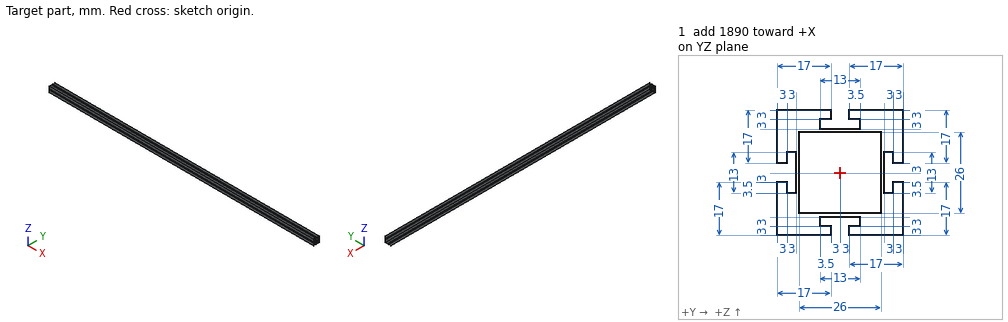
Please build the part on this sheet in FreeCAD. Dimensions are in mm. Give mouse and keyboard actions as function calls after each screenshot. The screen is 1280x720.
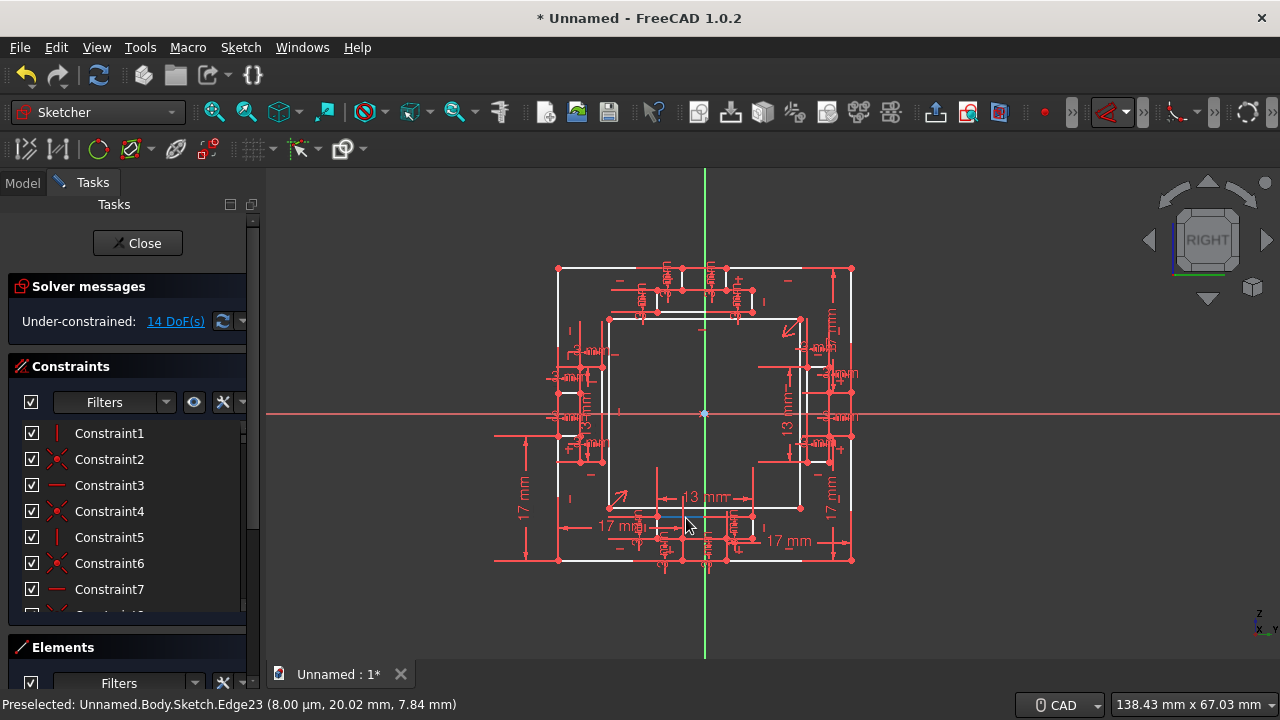
click(814, 268)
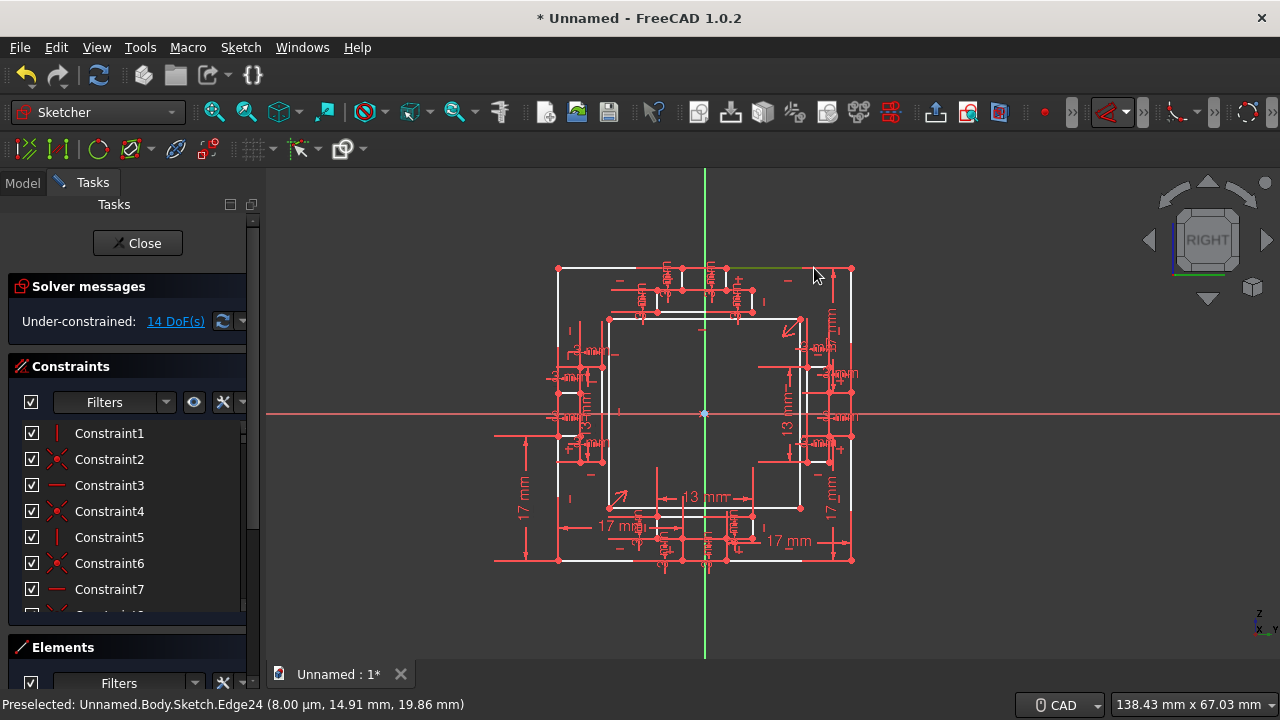
key(l)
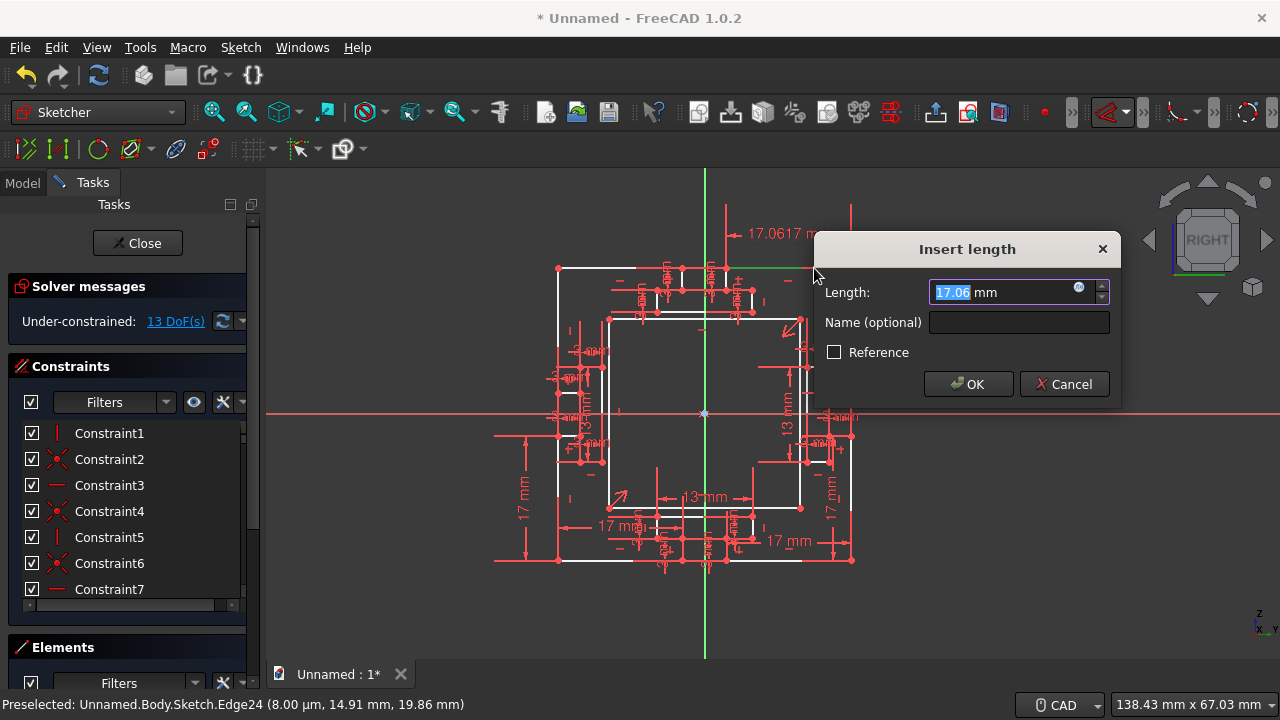
text(17)
key(Return)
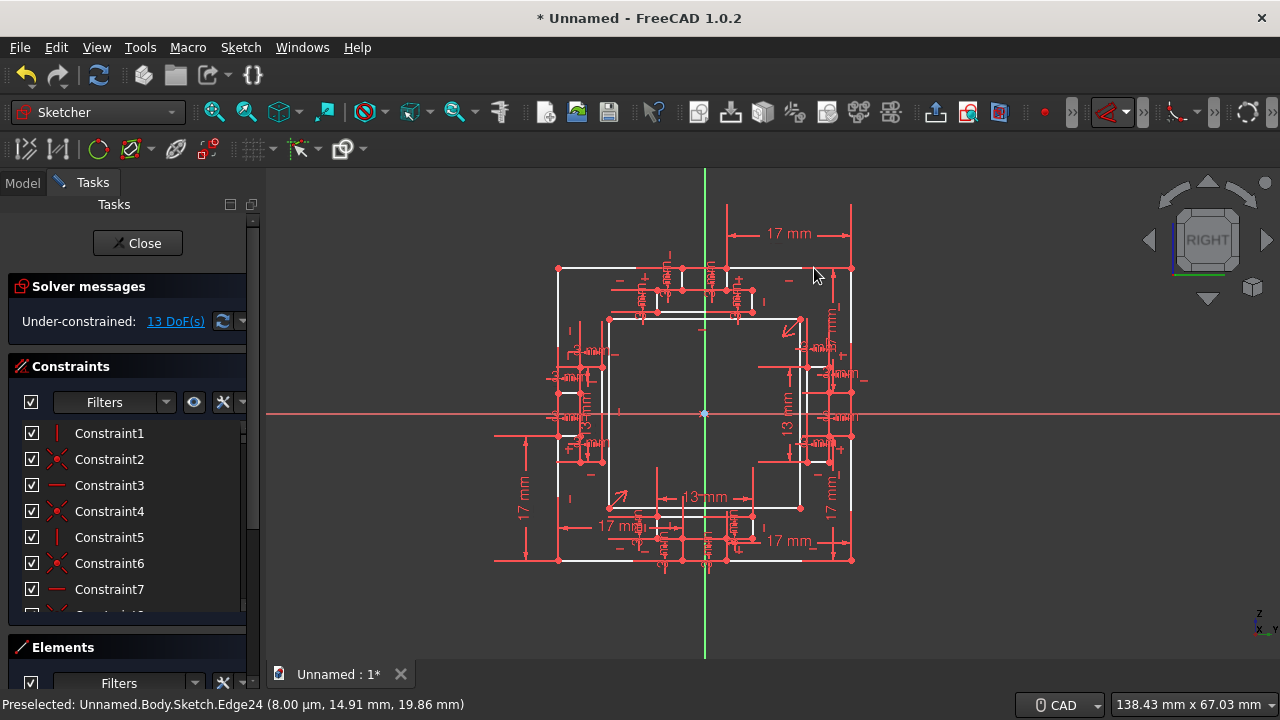
scroll(724, 312, up, 4)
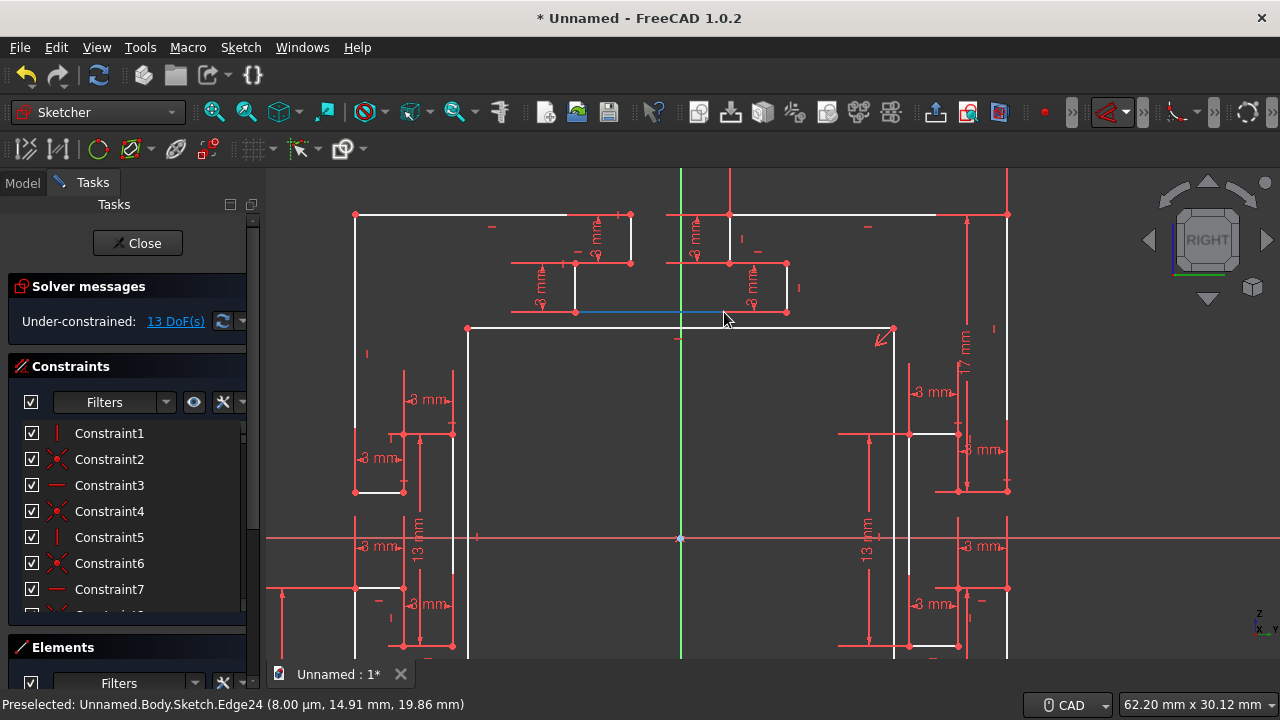
click(723, 312)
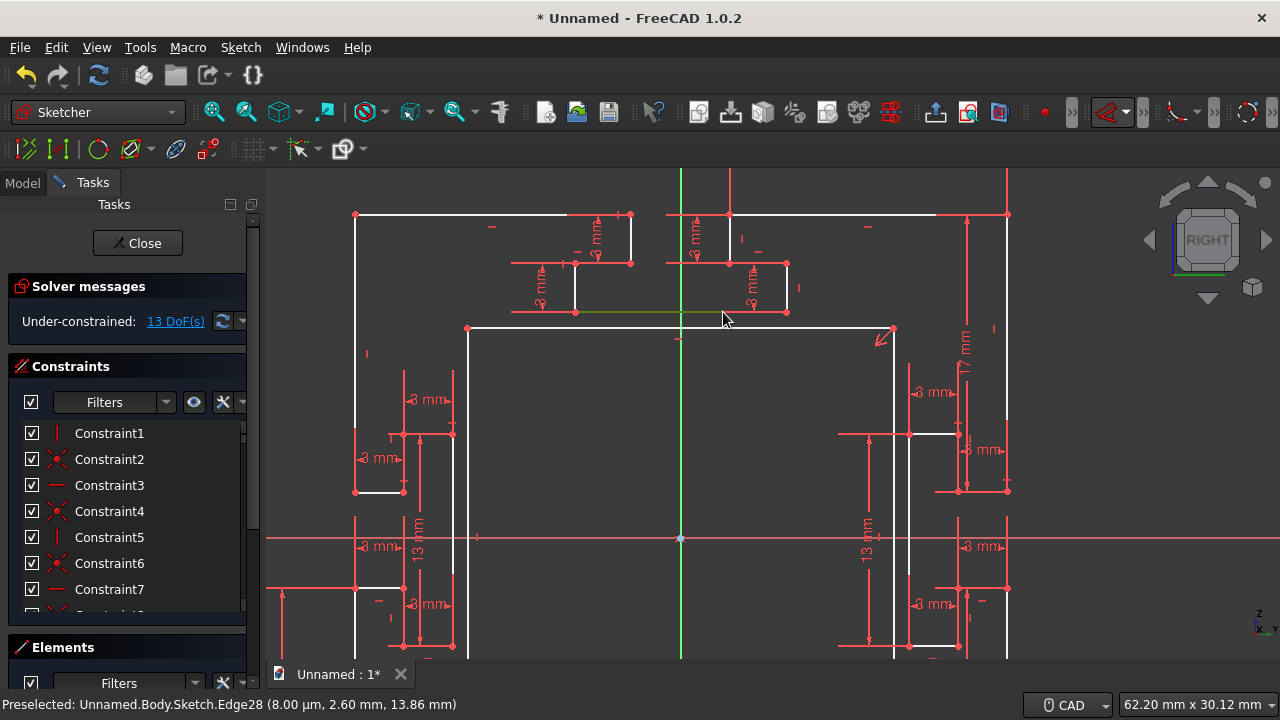
key(l)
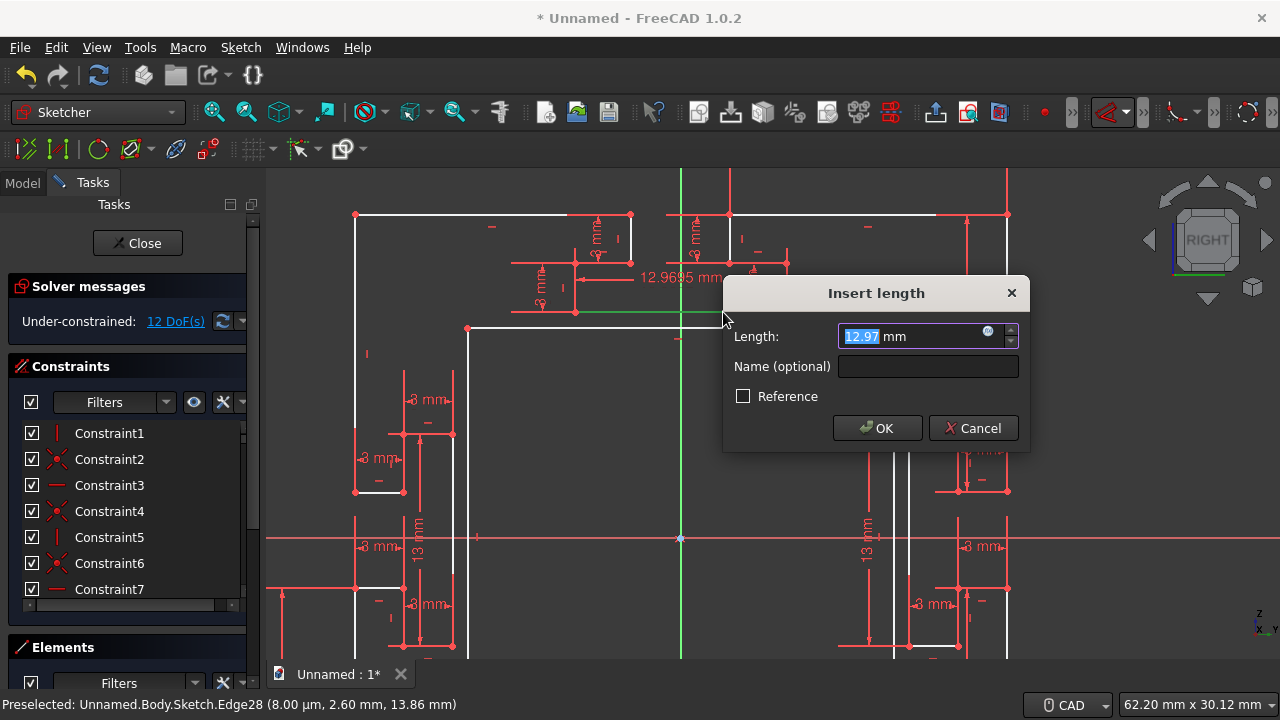
text(13)
key(Return)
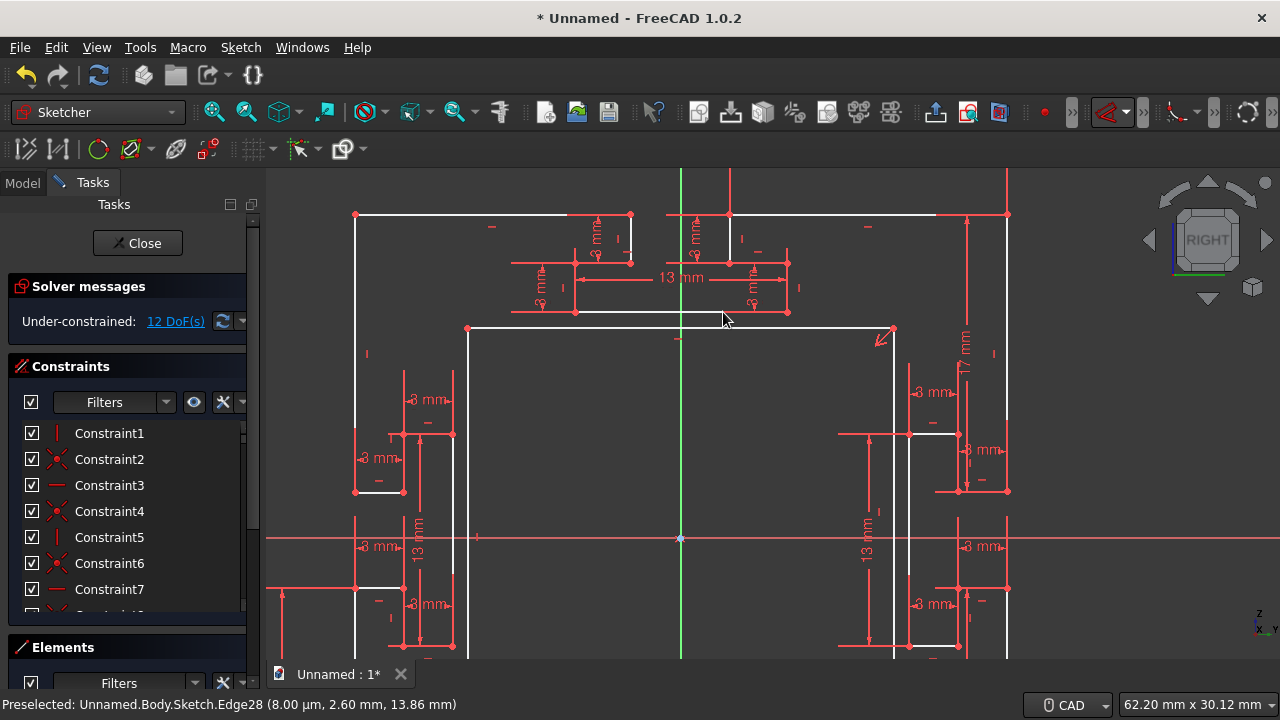
click(548, 215)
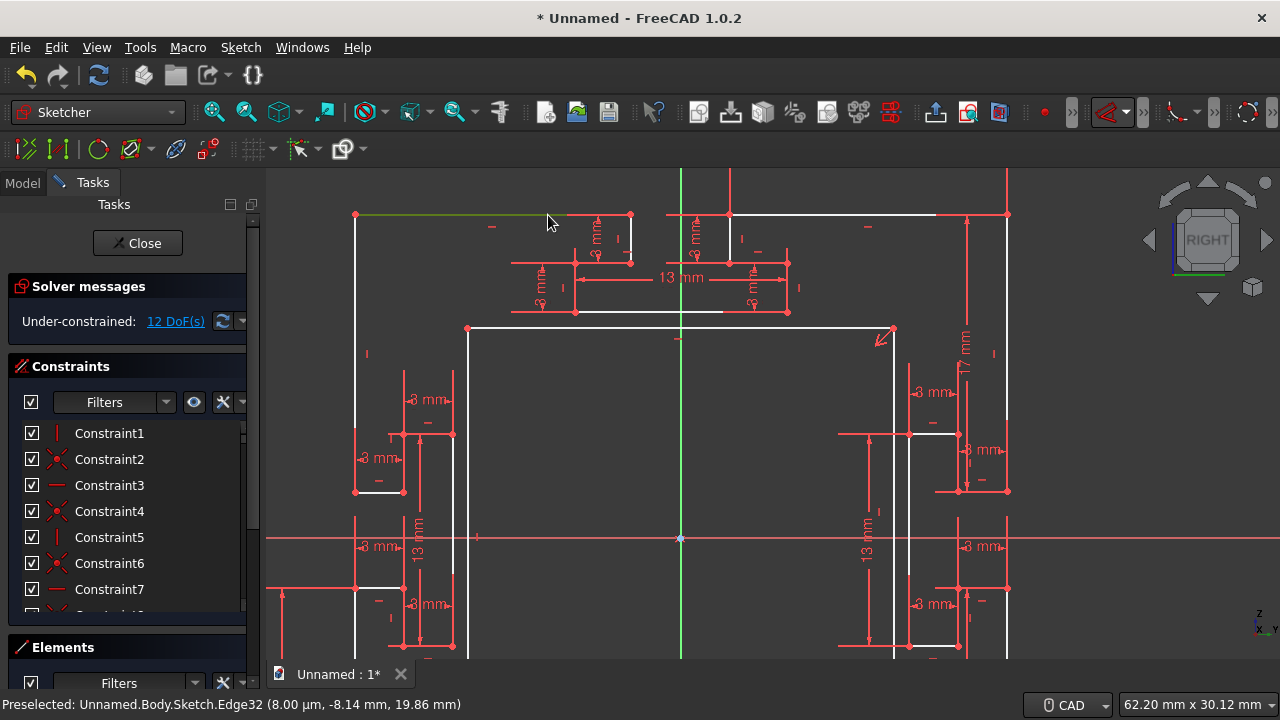
key(l)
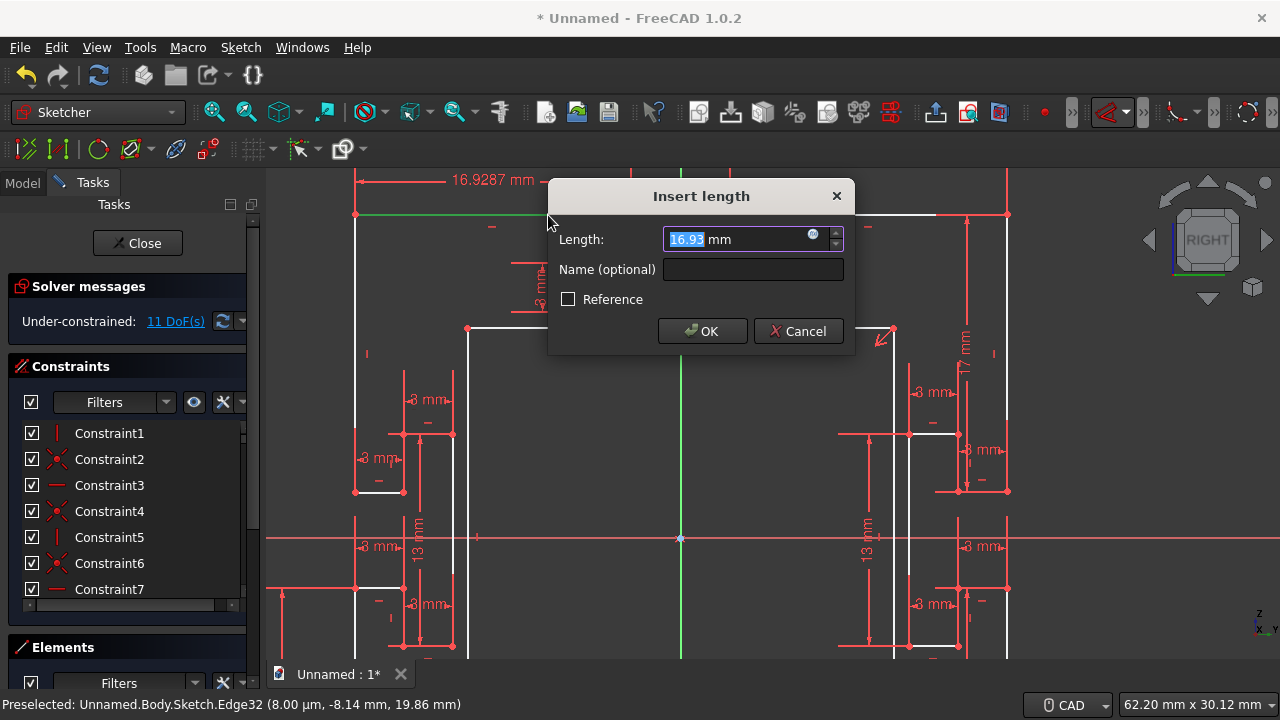
text(17)
key(Return)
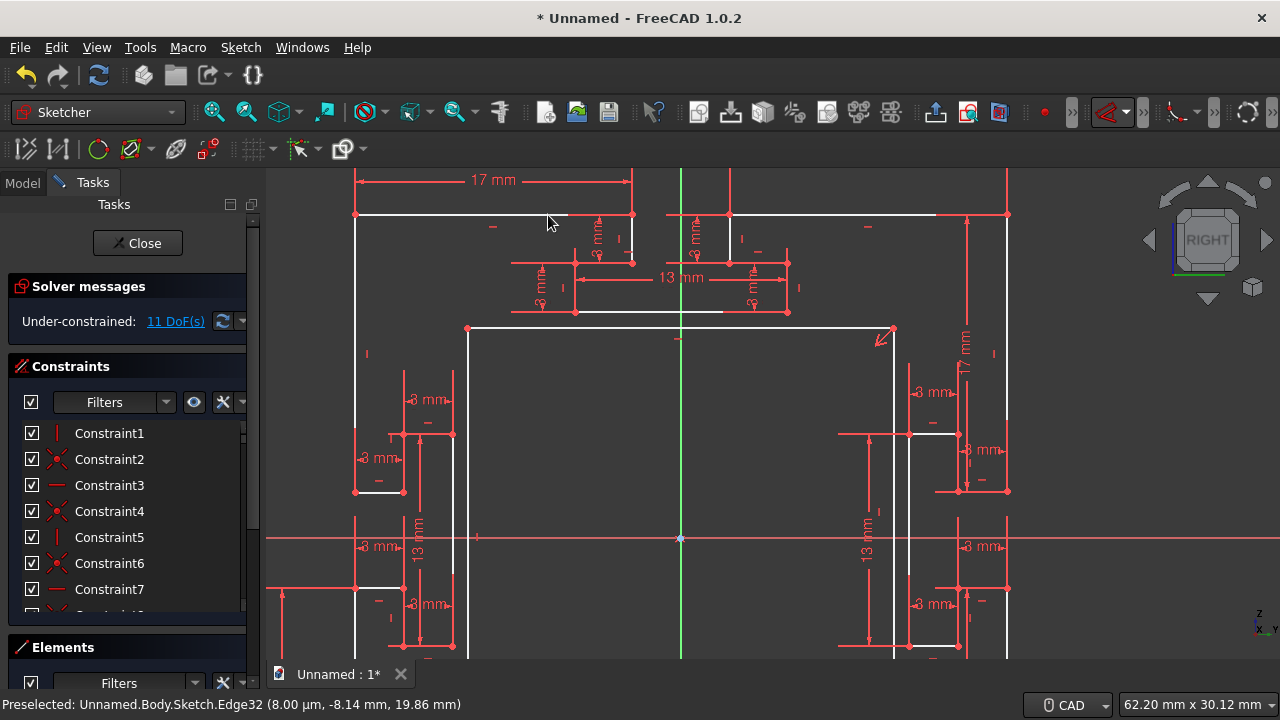
click(355, 298)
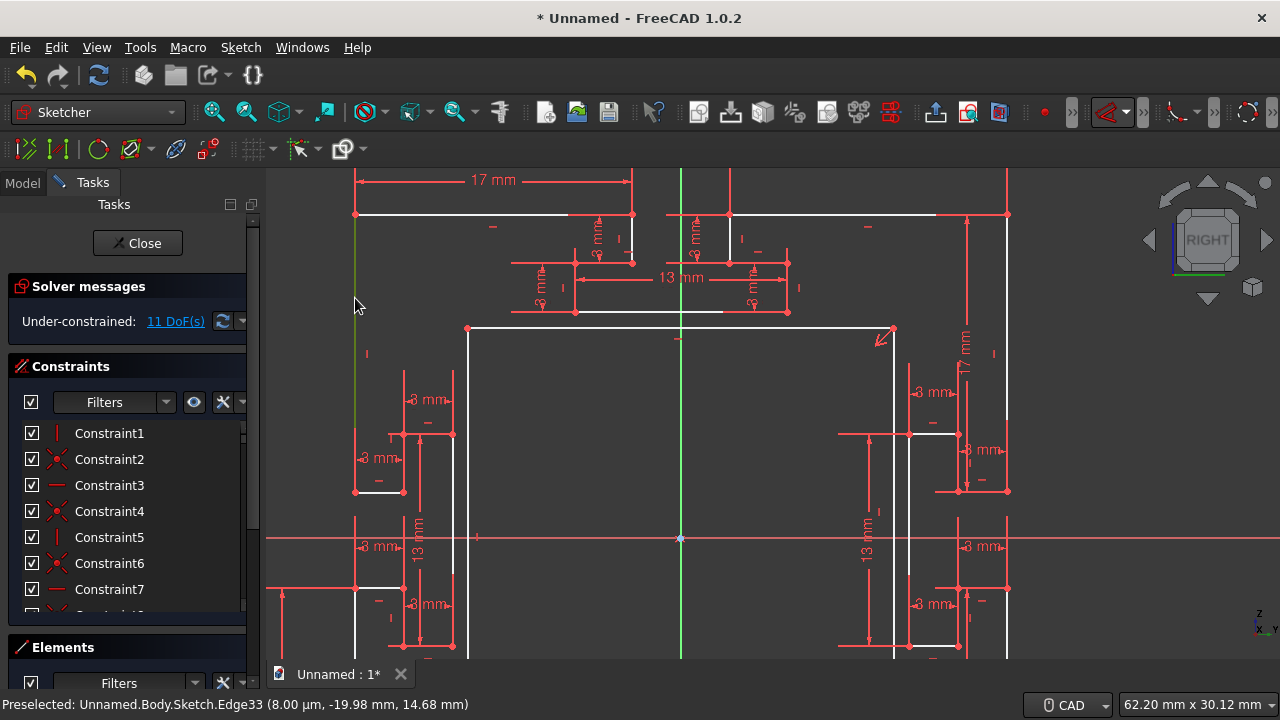
key(i)